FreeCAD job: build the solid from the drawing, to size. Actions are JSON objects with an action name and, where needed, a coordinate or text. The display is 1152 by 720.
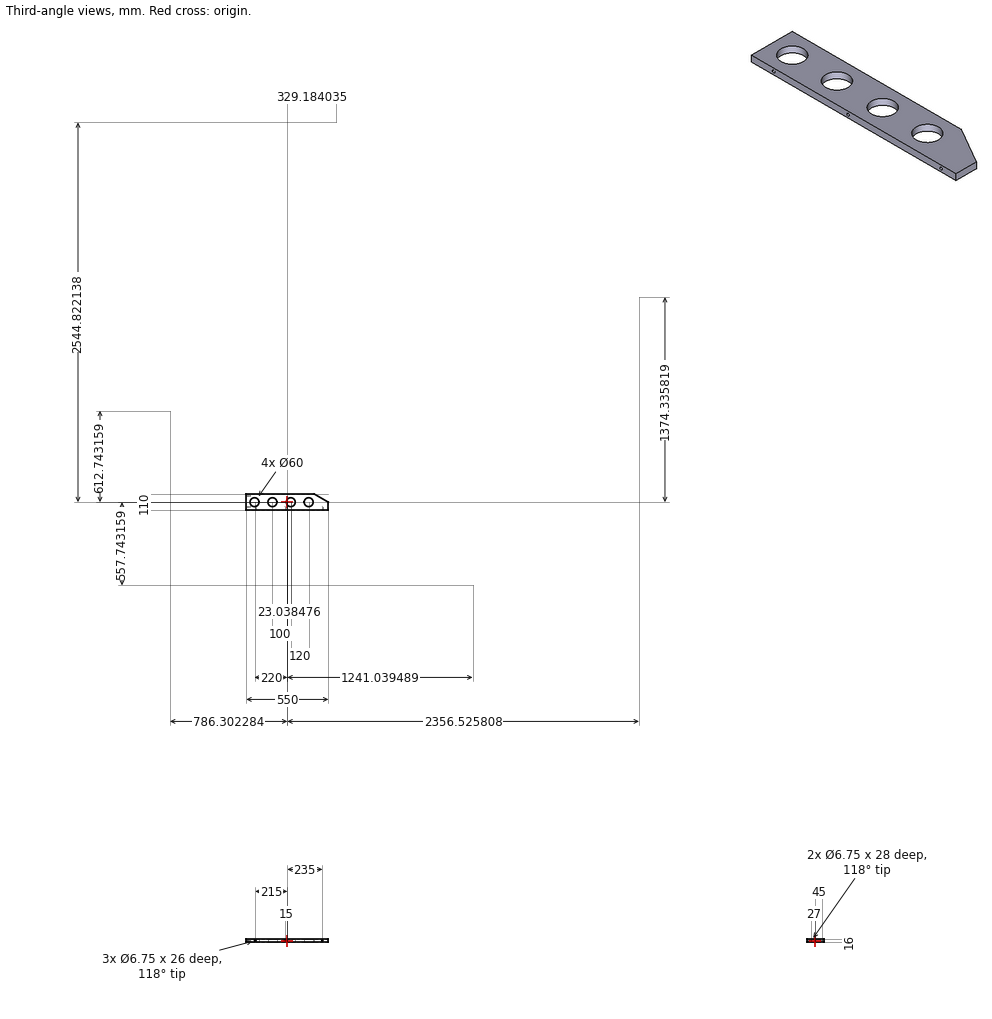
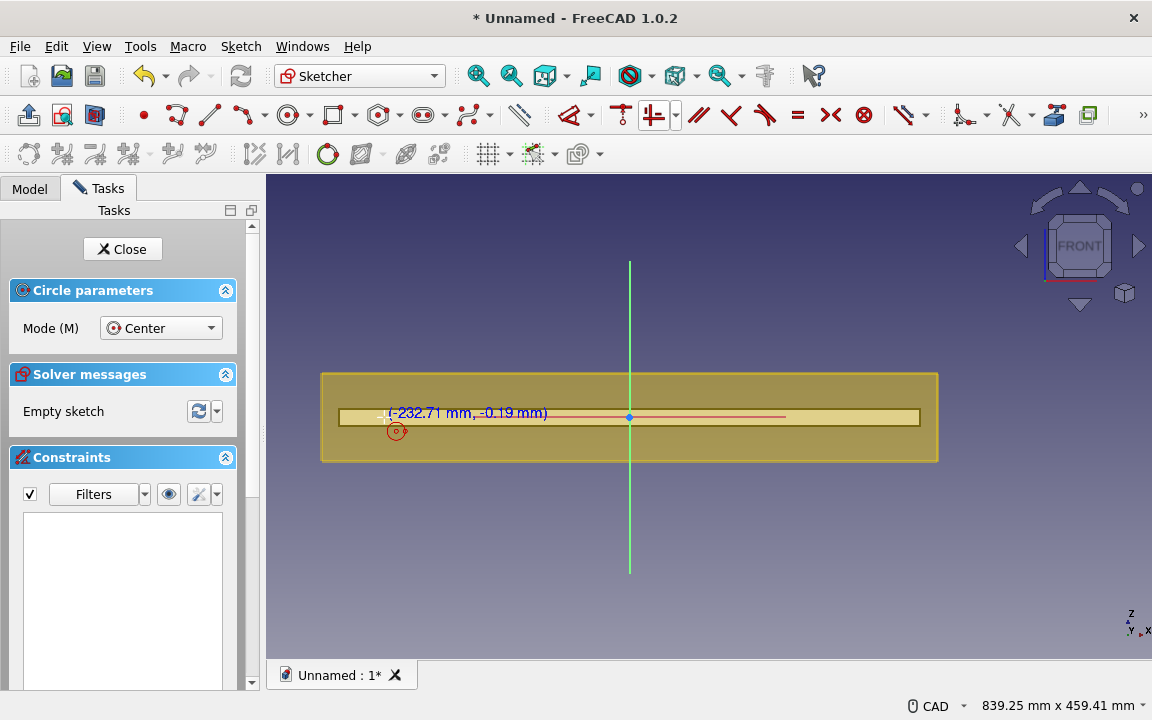
{"action": "left_click", "coordinate": [403, 417]}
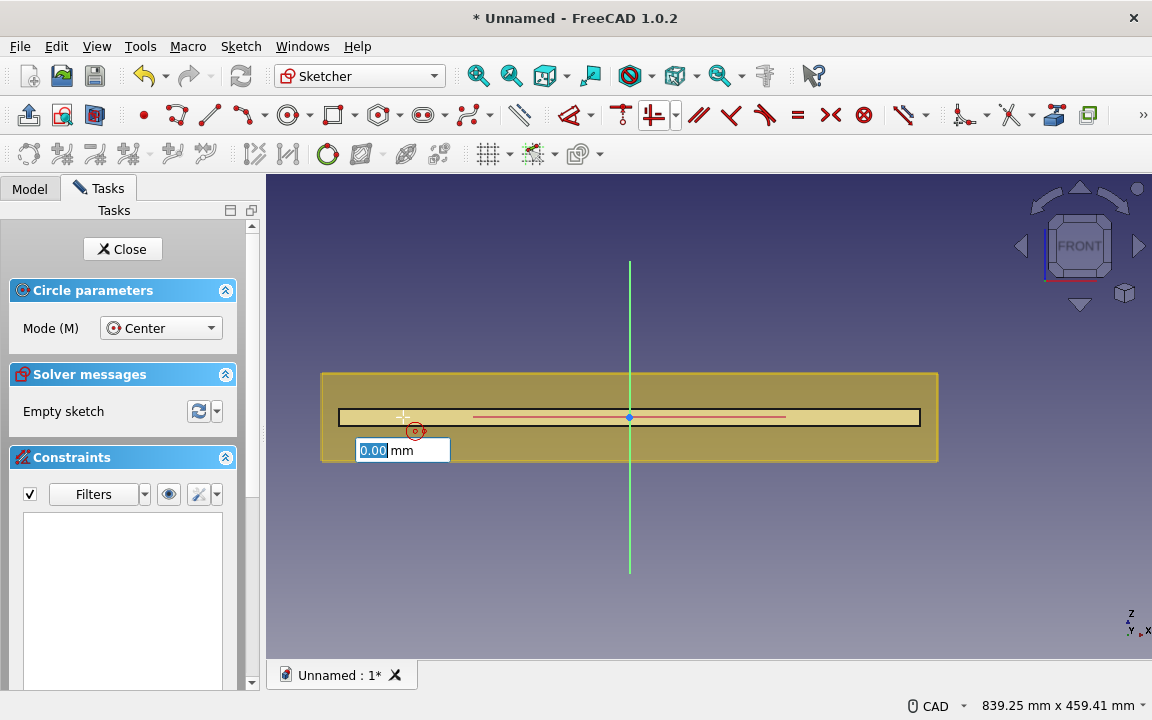
{"action": "scroll", "coordinate": [402, 421], "scroll_direction": "up", "scroll_amount": 8}
{"action": "mouse_move", "coordinate": [399, 418]}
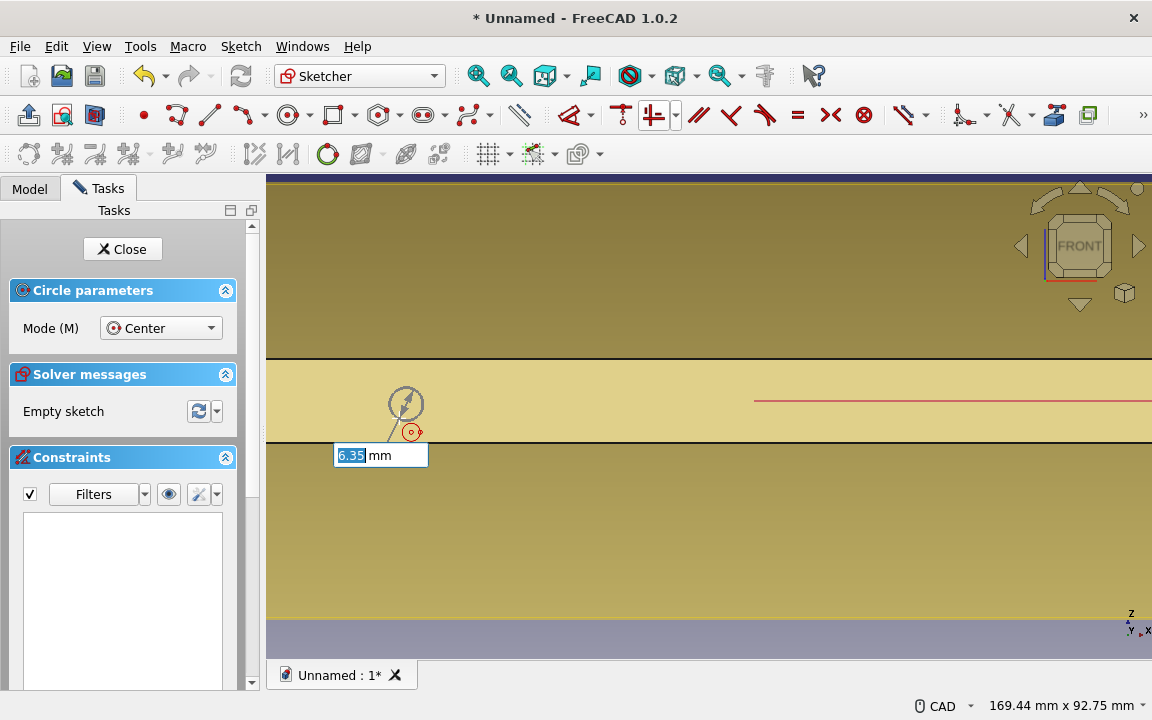
{"action": "type", "text": "6.75"}
{"action": "key", "text": "Return"}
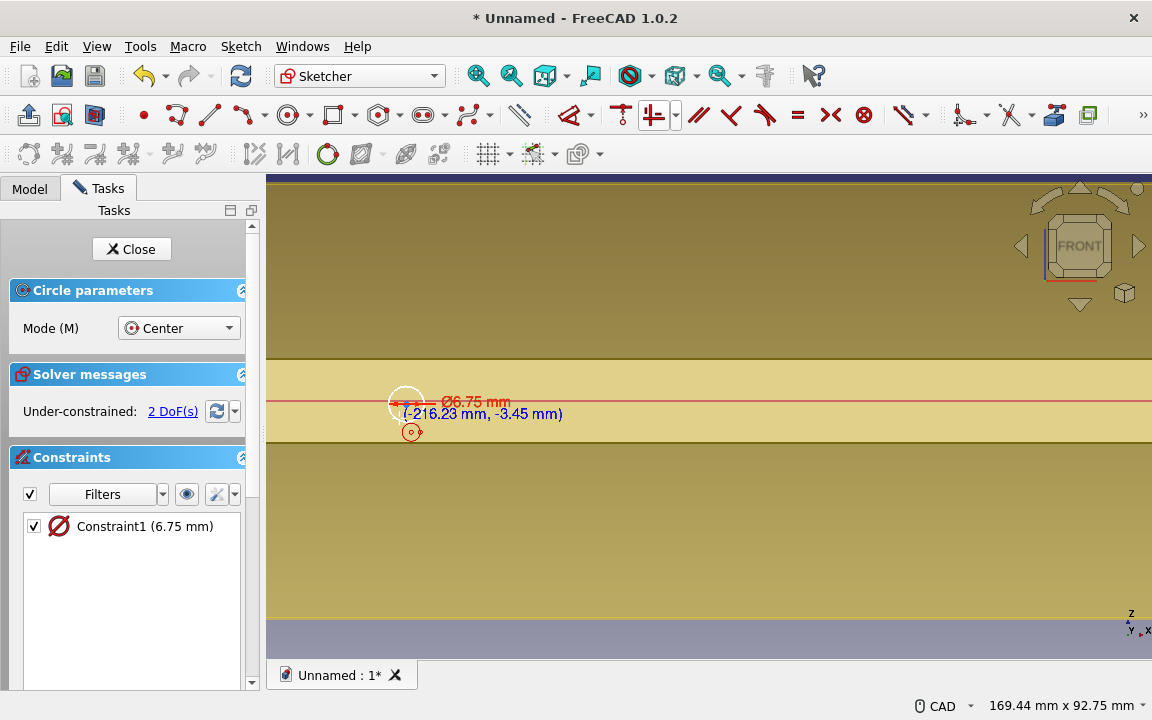
{"action": "scroll", "coordinate": [402, 420], "scroll_direction": "down", "scroll_amount": 8}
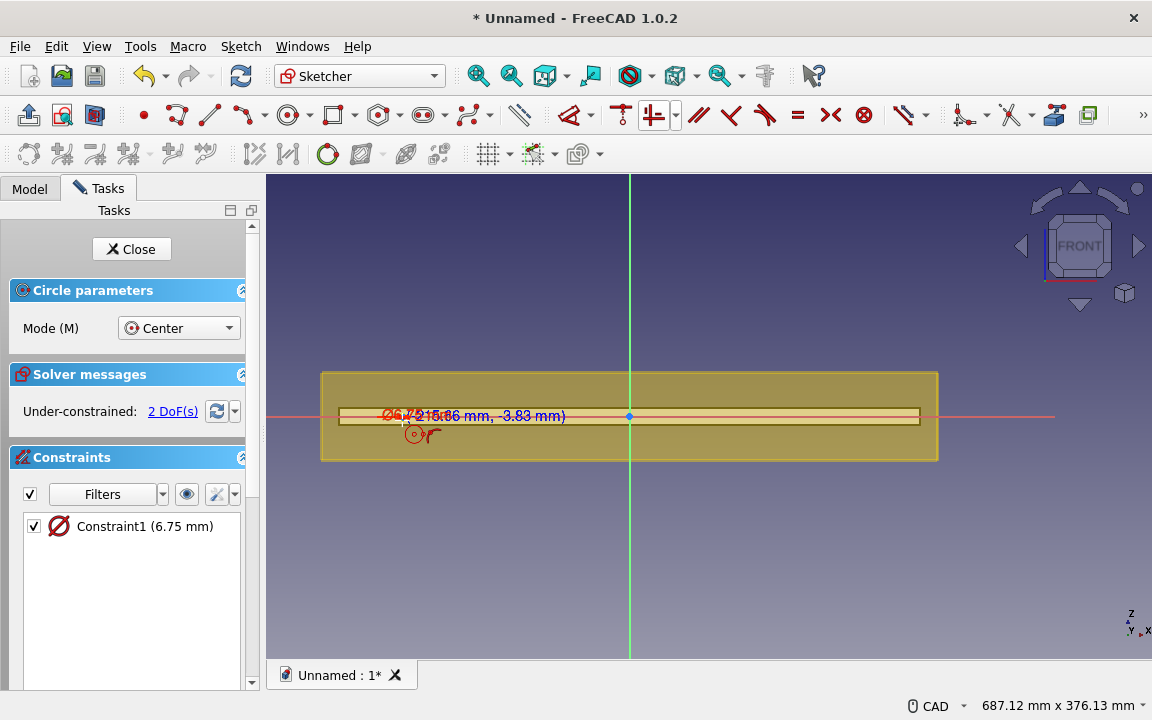
{"action": "scroll", "coordinate": [614, 417], "scroll_direction": "up", "scroll_amount": 10}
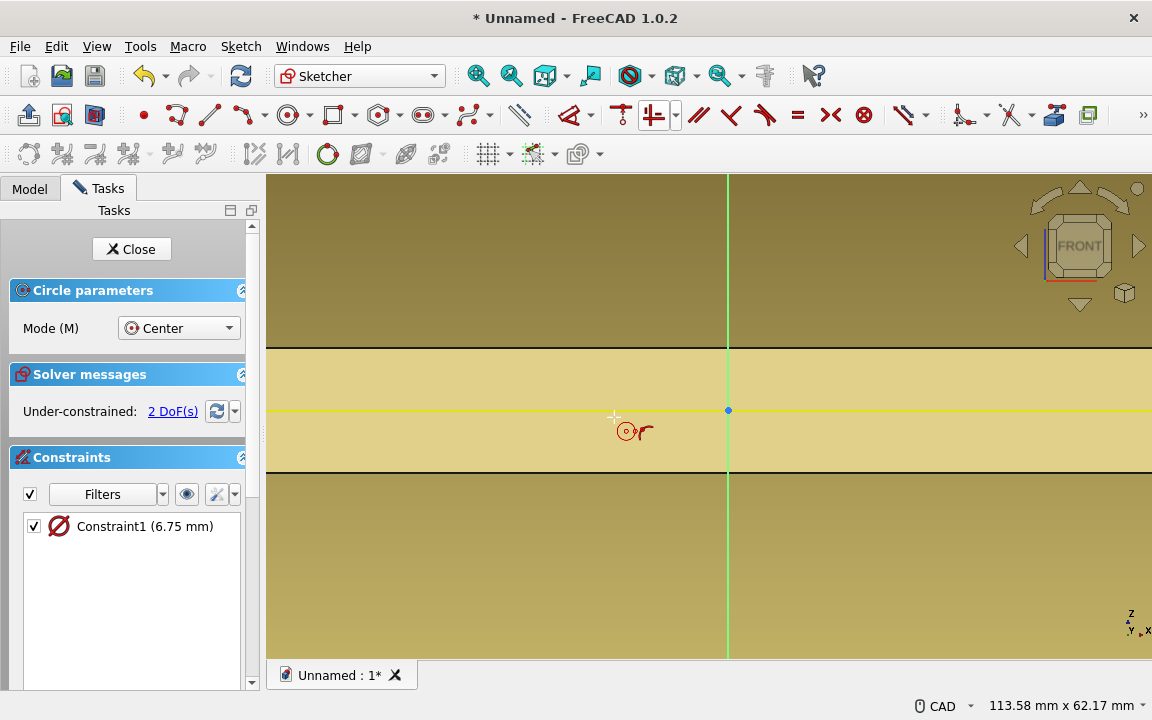
{"action": "scroll", "coordinate": [615, 417], "scroll_direction": "down", "scroll_amount": 10}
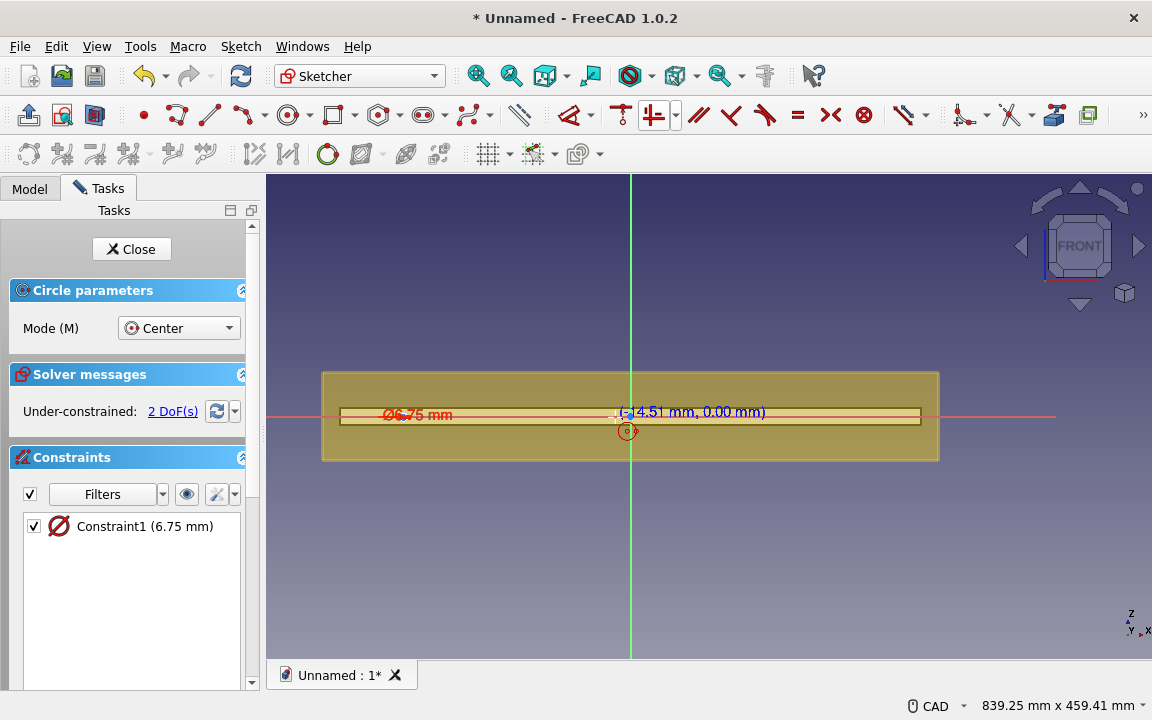
{"action": "left_click", "coordinate": [615, 417]}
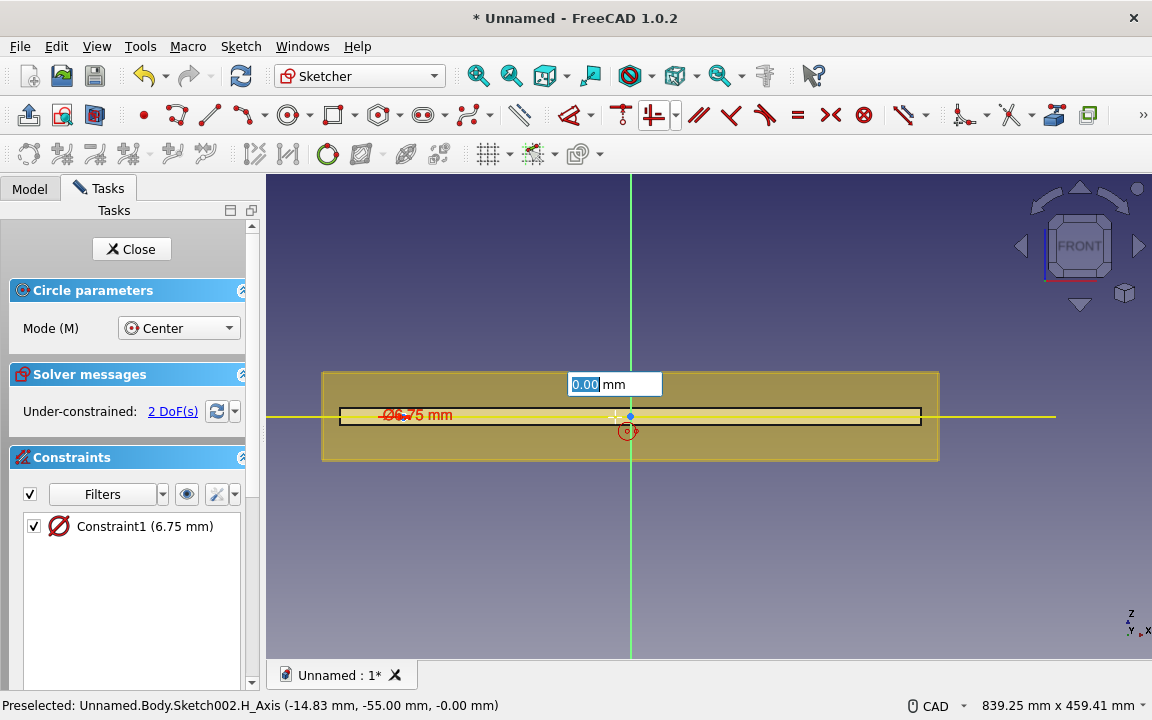
{"action": "scroll", "coordinate": [614, 420], "scroll_direction": "up", "scroll_amount": 8}
{"action": "mouse_move", "coordinate": [610, 418]}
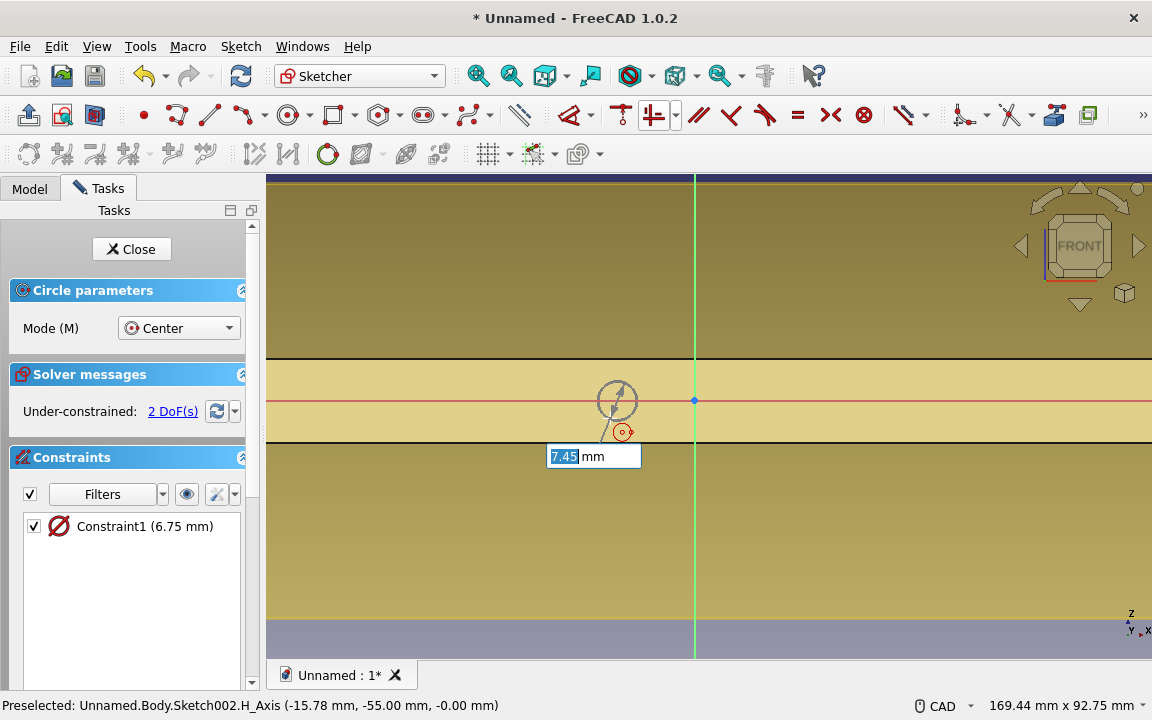
{"action": "type", "text": "6.75"}
{"action": "key", "text": "Return"}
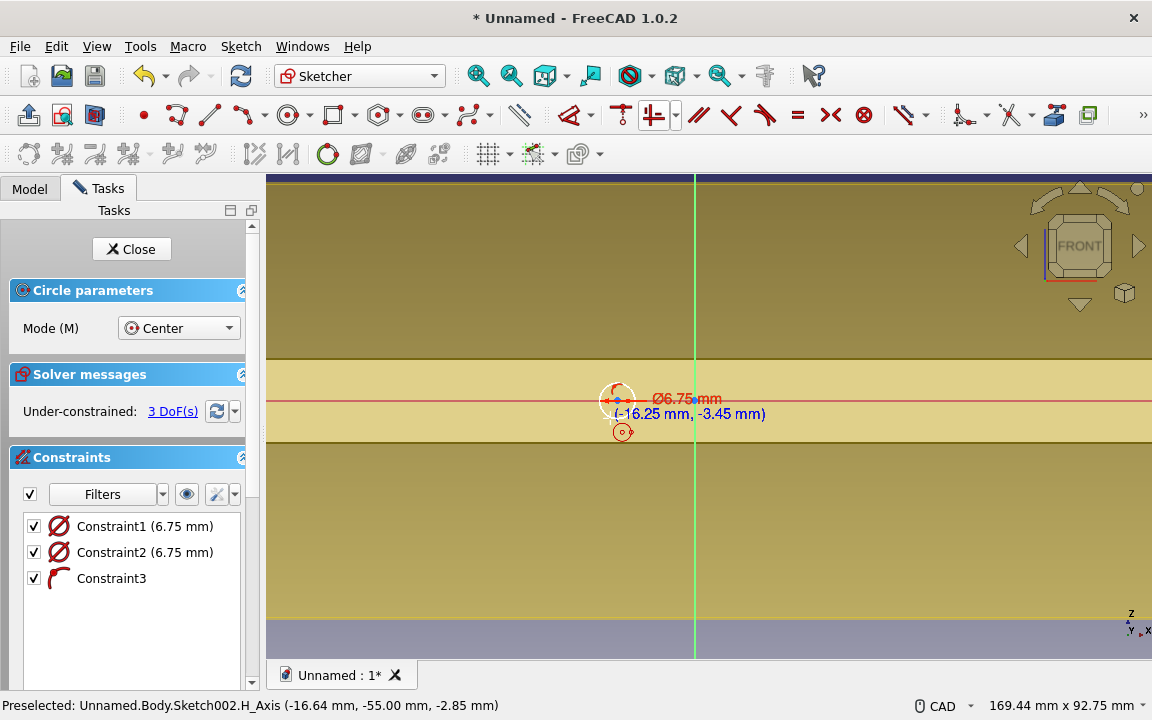
{"action": "scroll", "coordinate": [613, 420], "scroll_direction": "down", "scroll_amount": 8}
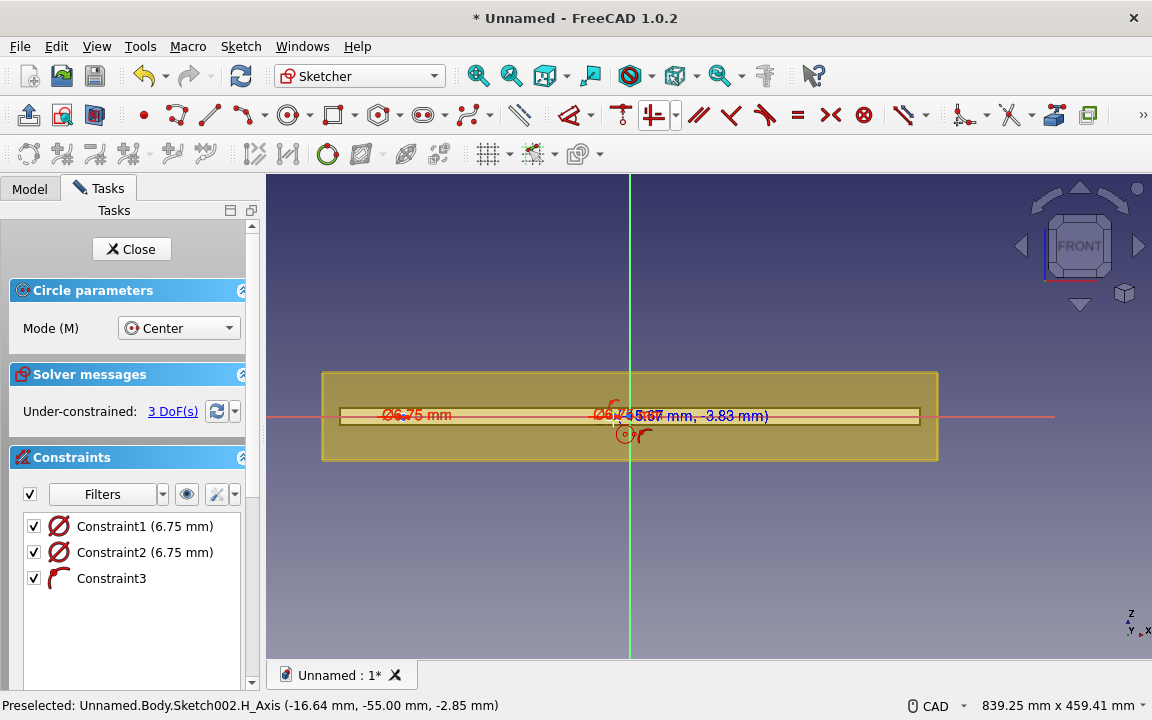
{"action": "scroll", "coordinate": [878, 417], "scroll_direction": "up", "scroll_amount": 10}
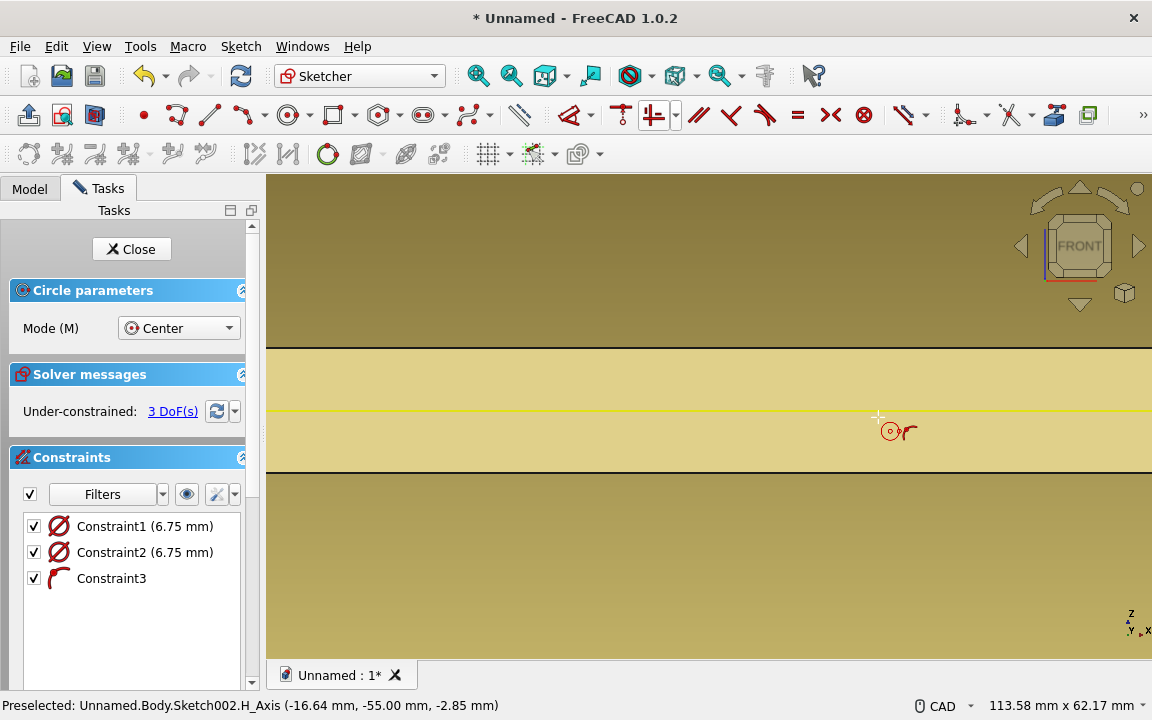
{"action": "scroll", "coordinate": [879, 417], "scroll_direction": "down", "scroll_amount": 10}